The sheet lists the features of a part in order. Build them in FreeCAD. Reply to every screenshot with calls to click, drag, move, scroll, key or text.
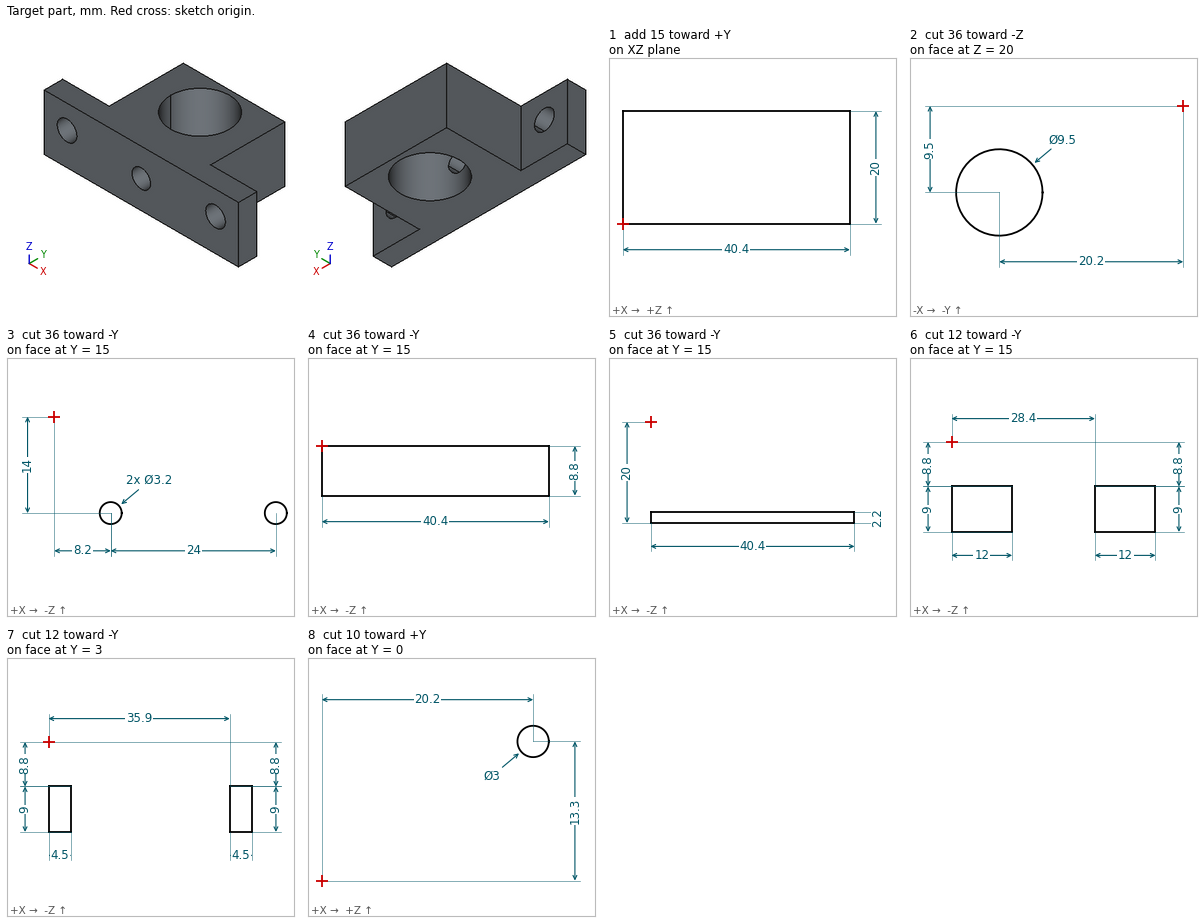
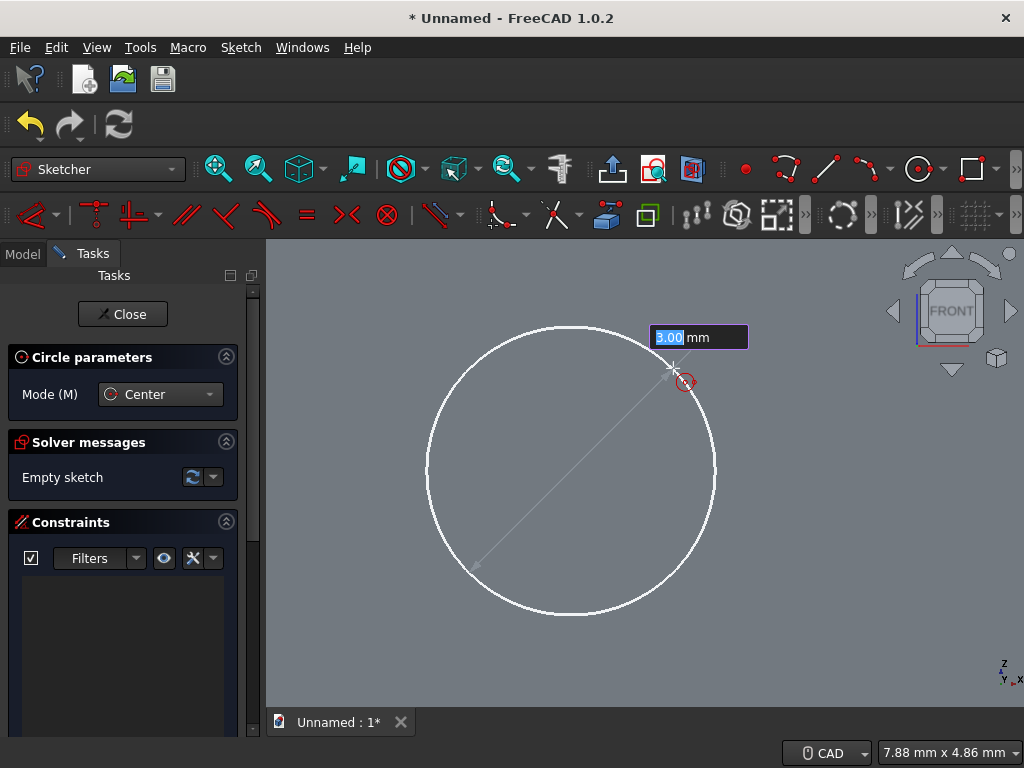
text(3)
key(Return)
key(Escape)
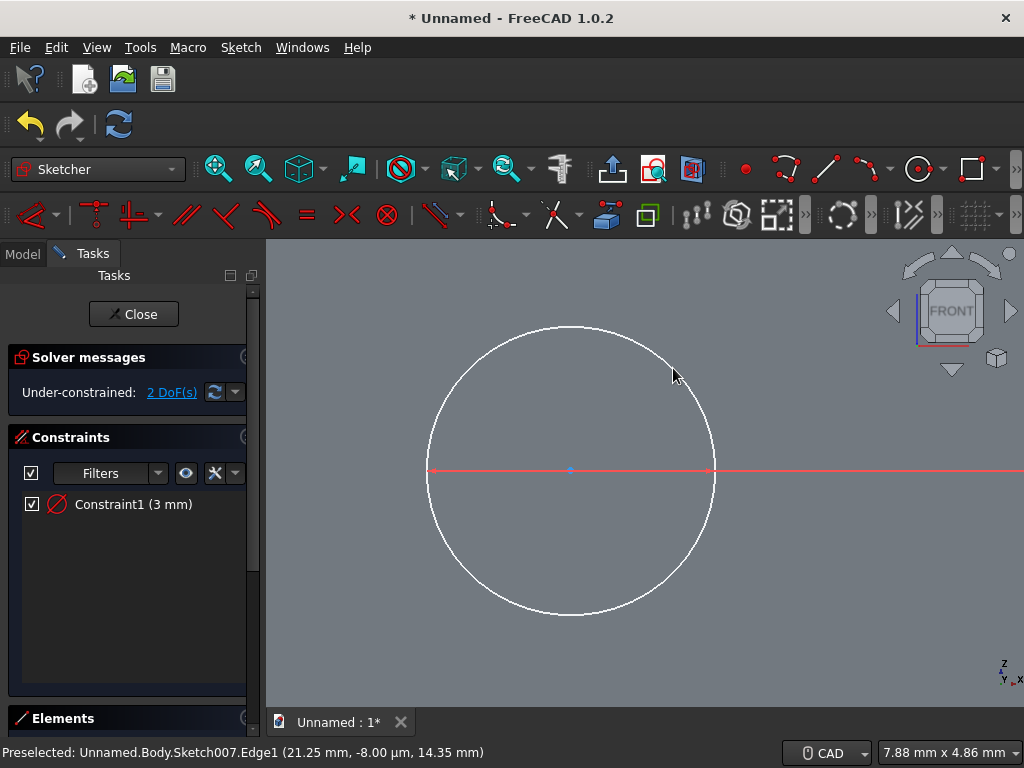
click(571, 471)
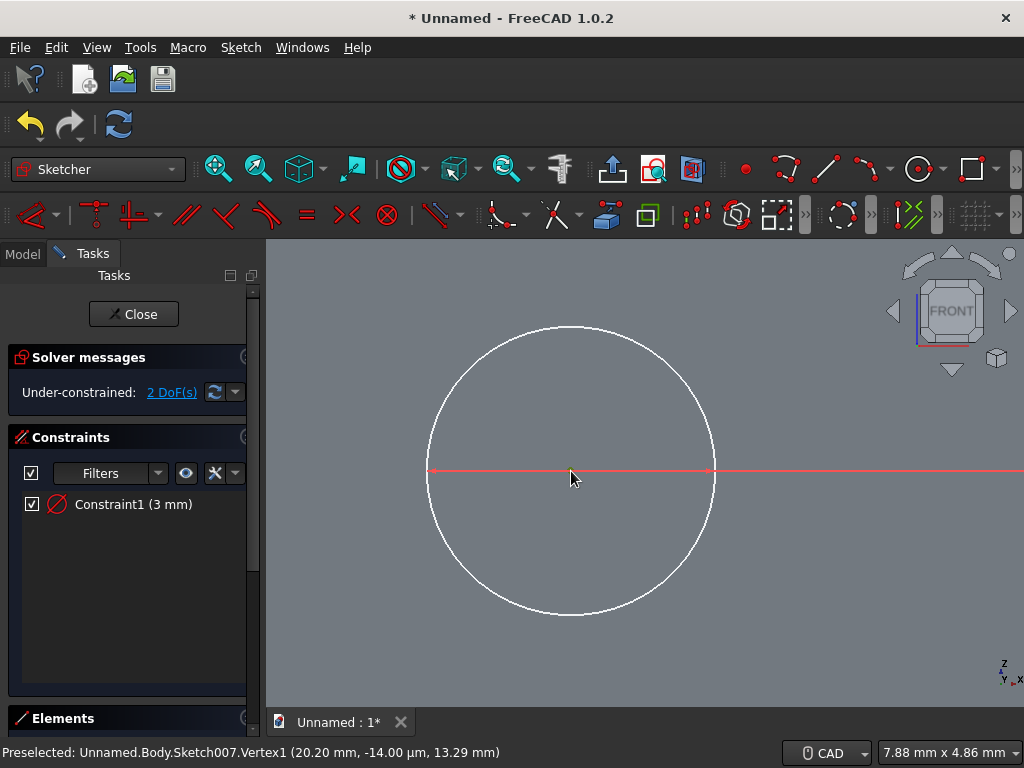
key(l)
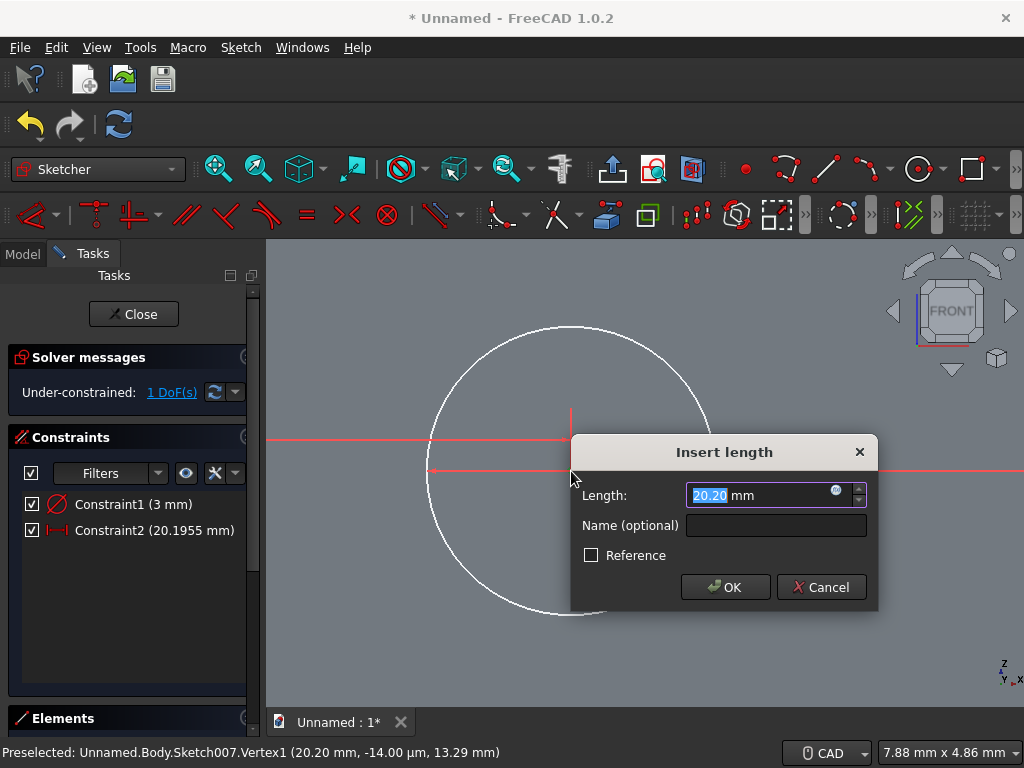
text(20.2)
key(Return)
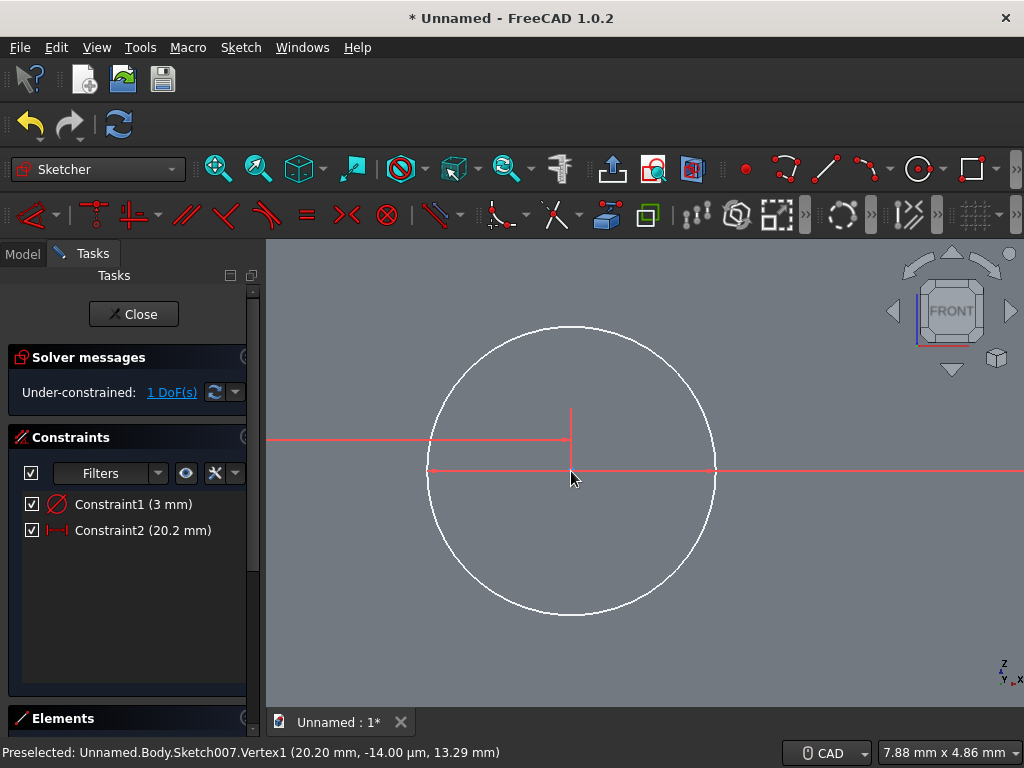
click(571, 471)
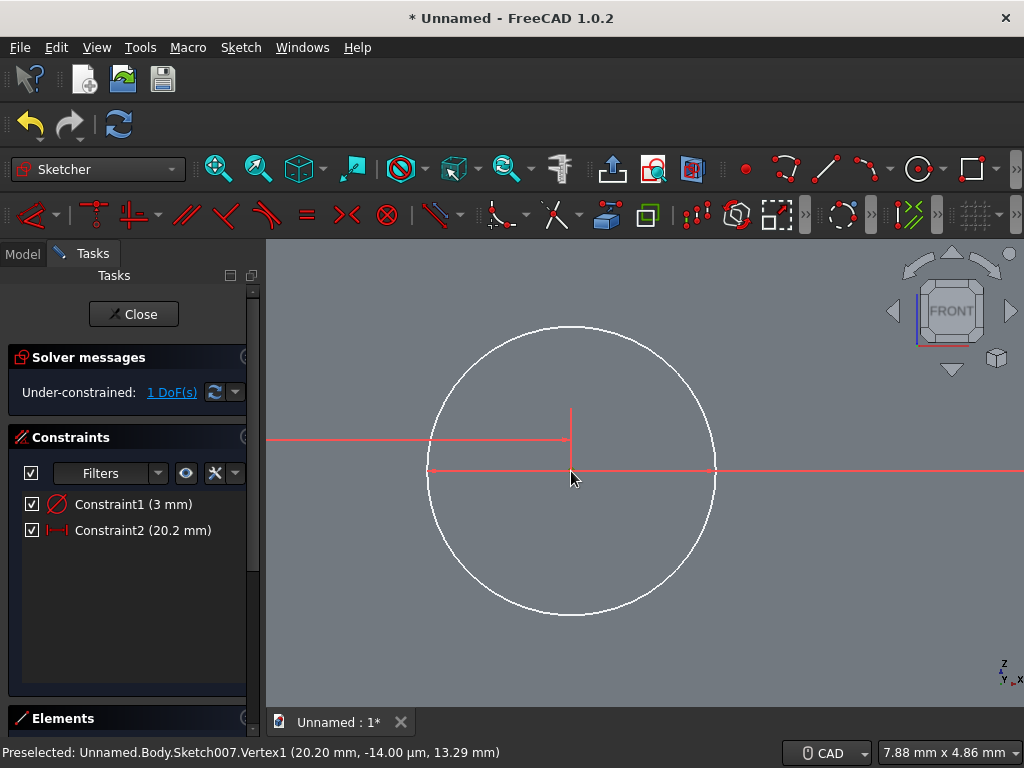
key(i)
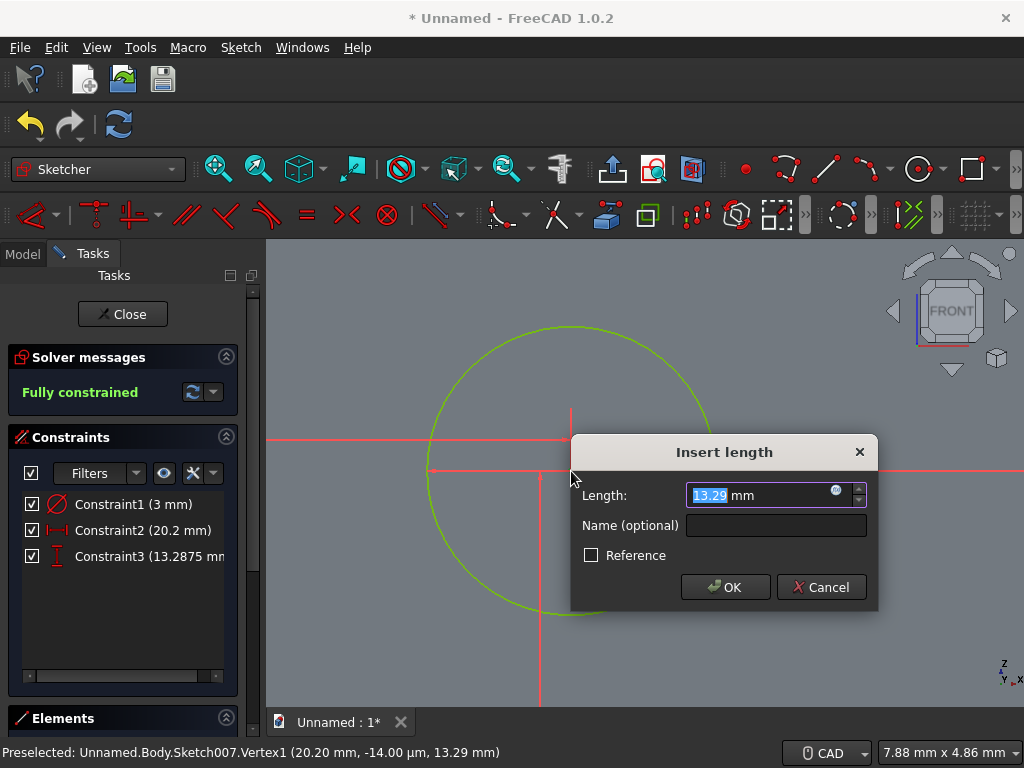
text(13.3)
key(Return)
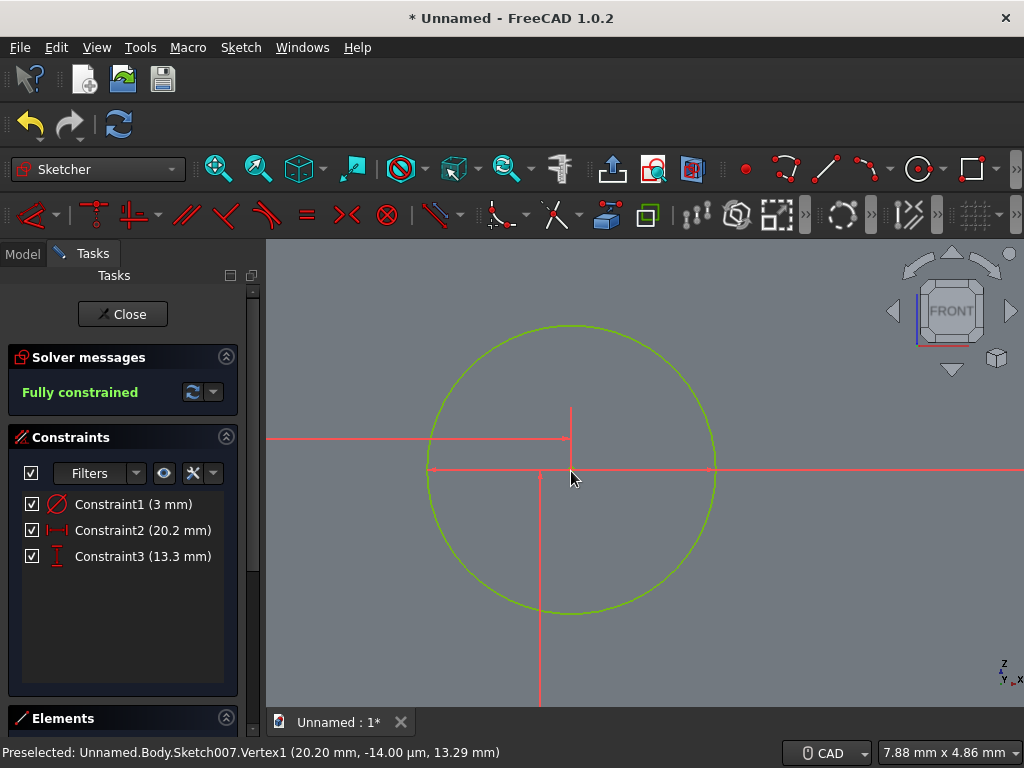
click(123, 314)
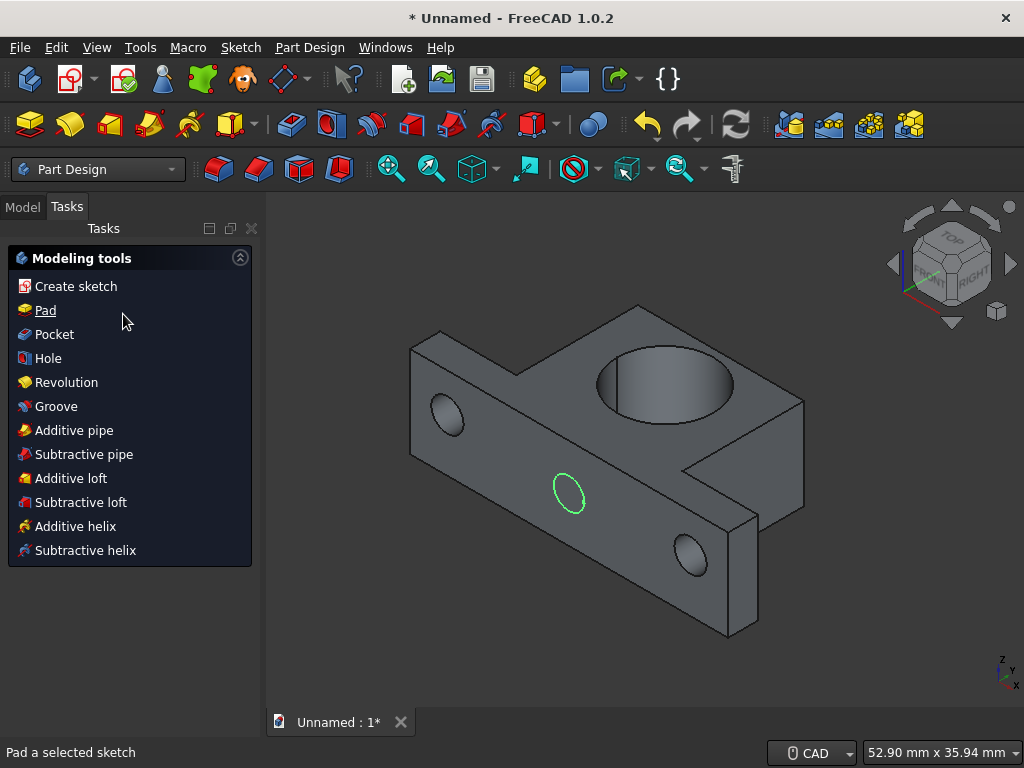
click(292, 124)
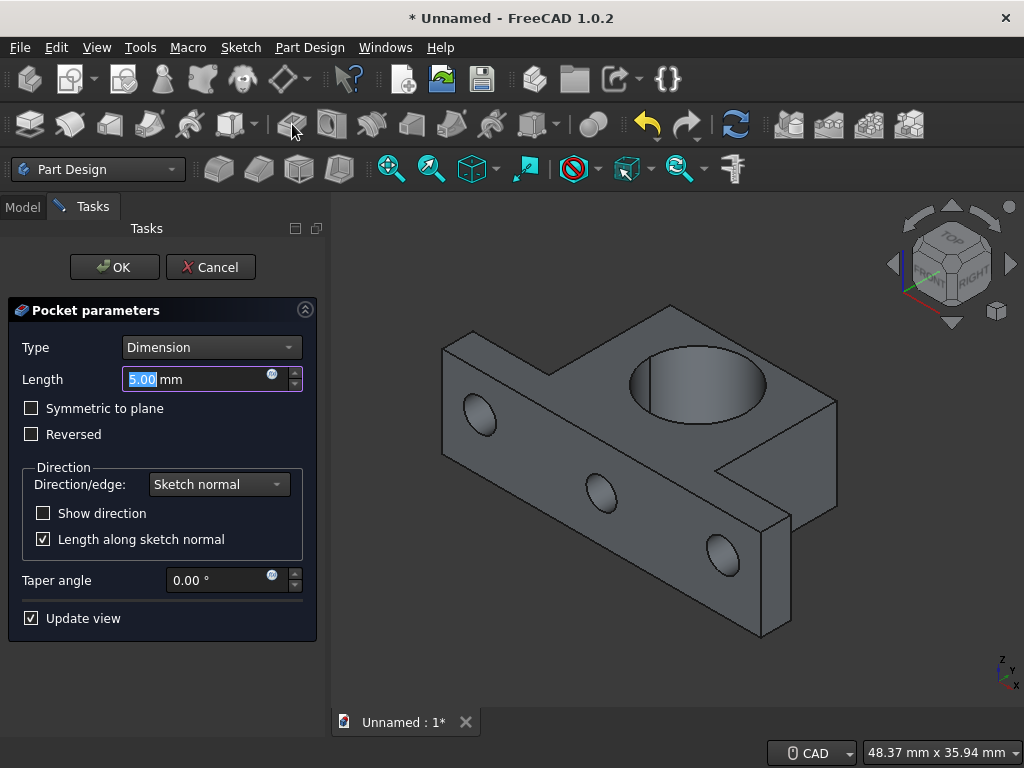
text(10)
key(Tab)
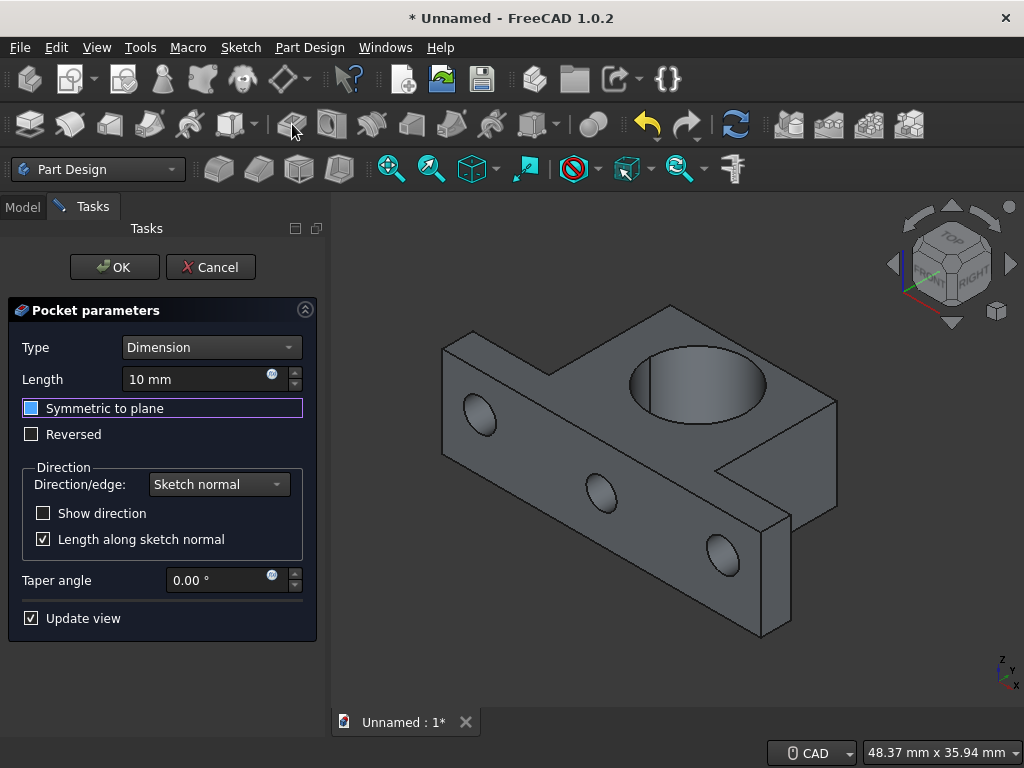
click(115, 267)